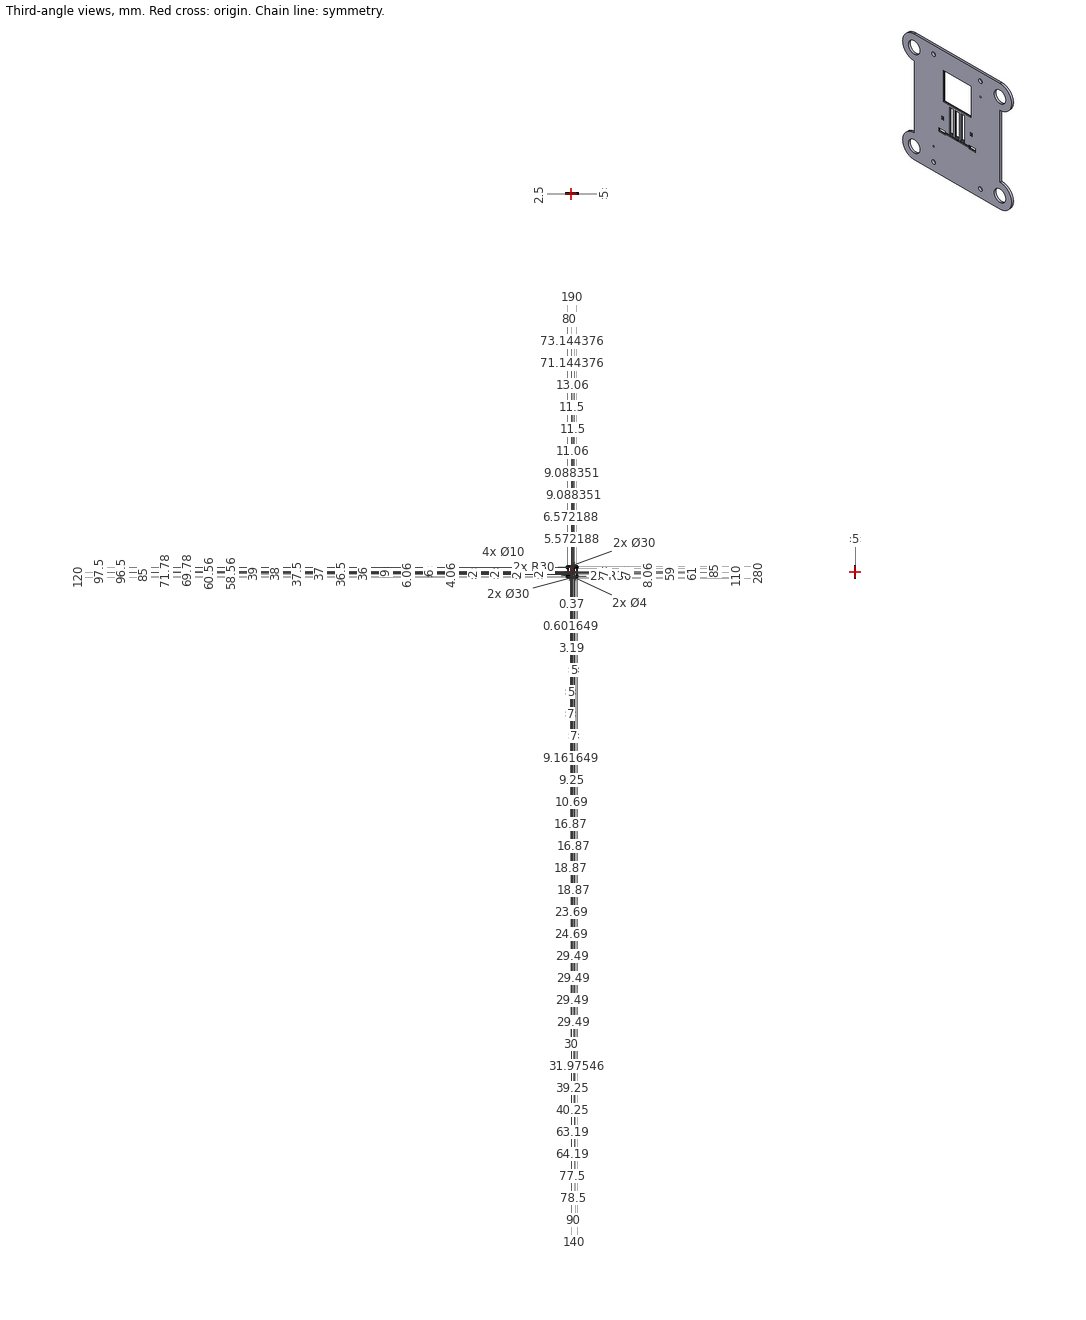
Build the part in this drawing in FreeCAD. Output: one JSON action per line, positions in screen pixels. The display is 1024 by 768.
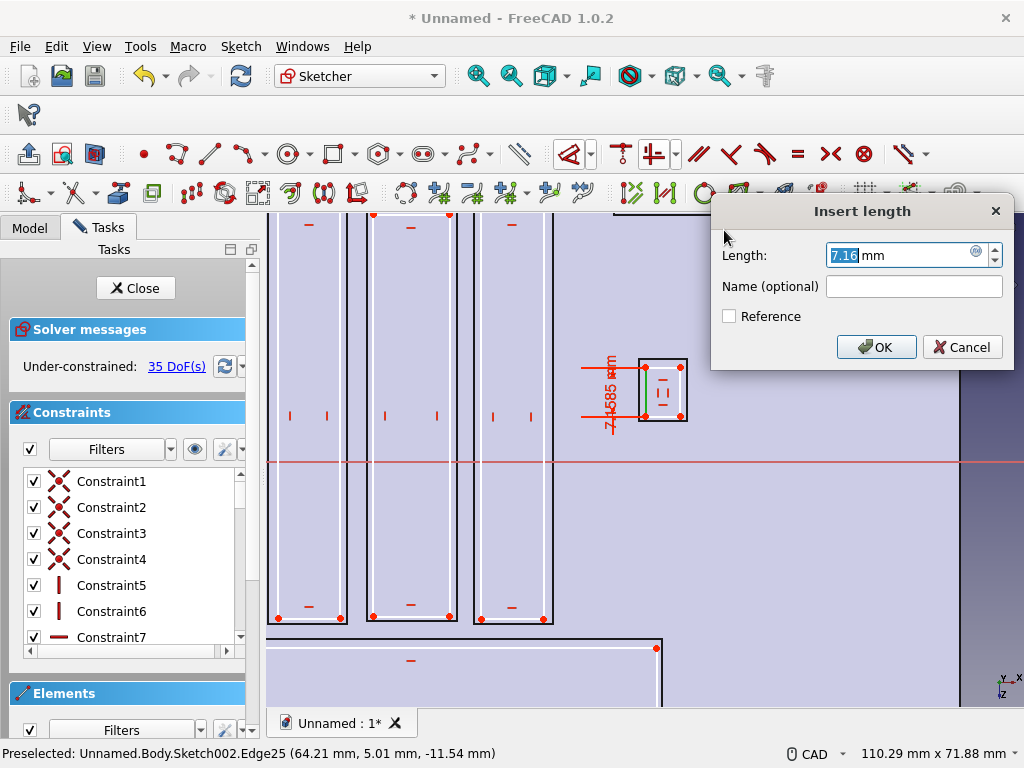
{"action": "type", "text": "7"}
{"action": "key", "text": "Return"}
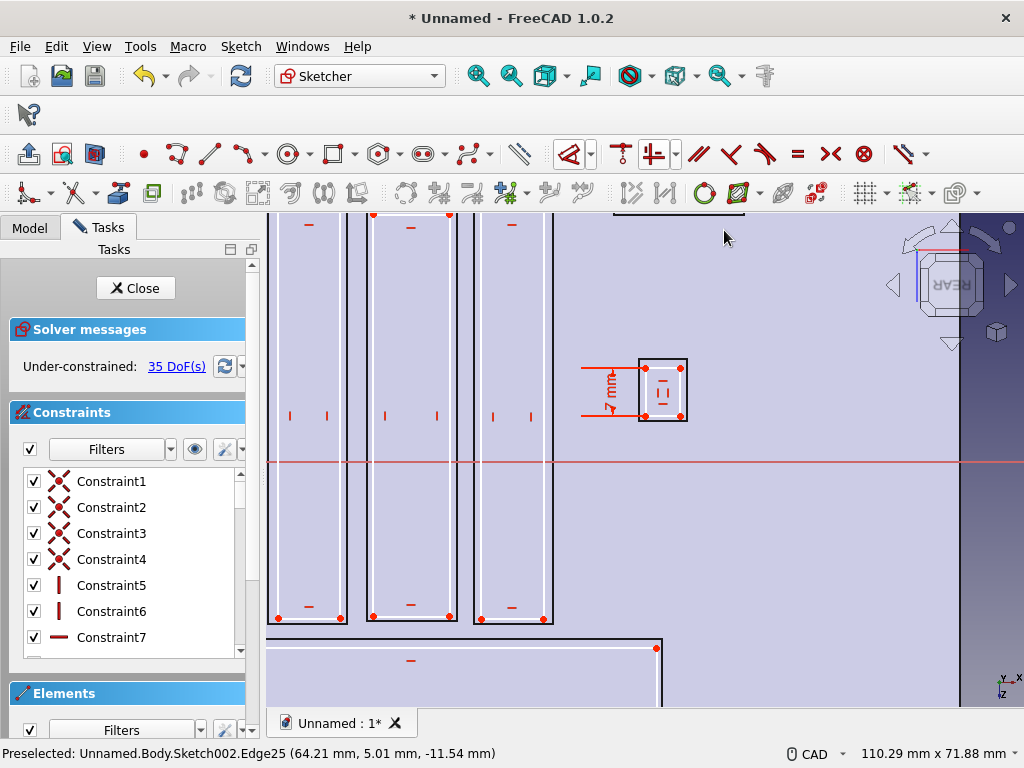
{"action": "scroll", "coordinate": [656, 416], "scroll_direction": "up", "scroll_amount": 2}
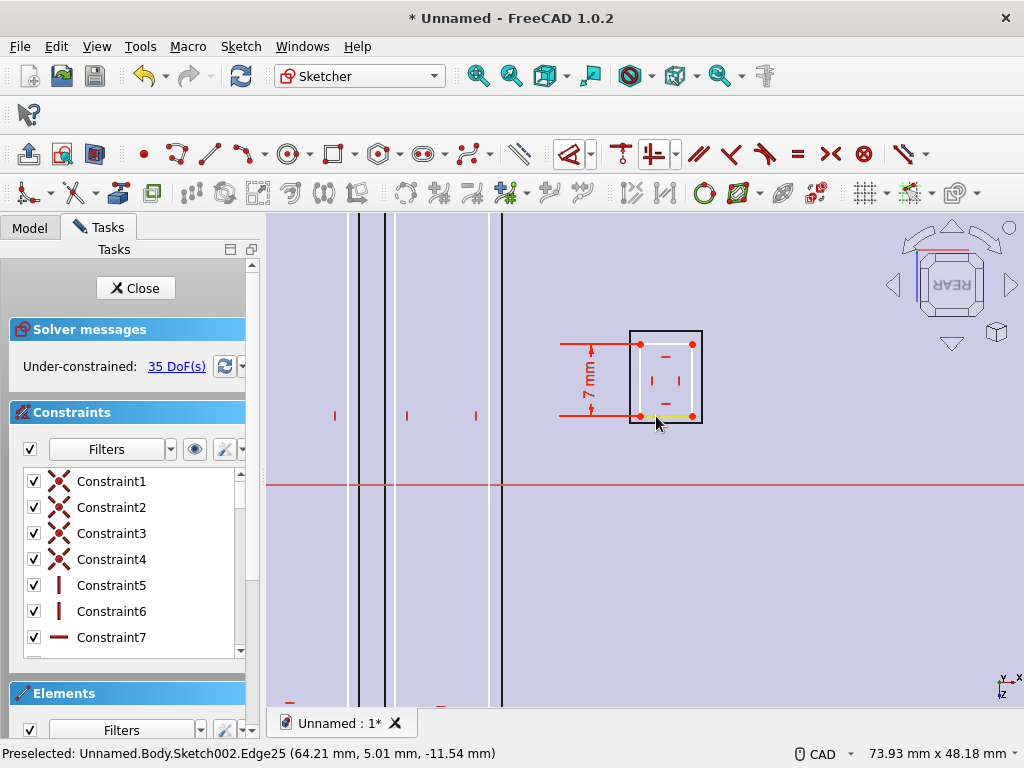
{"action": "left_click", "coordinate": [656, 416]}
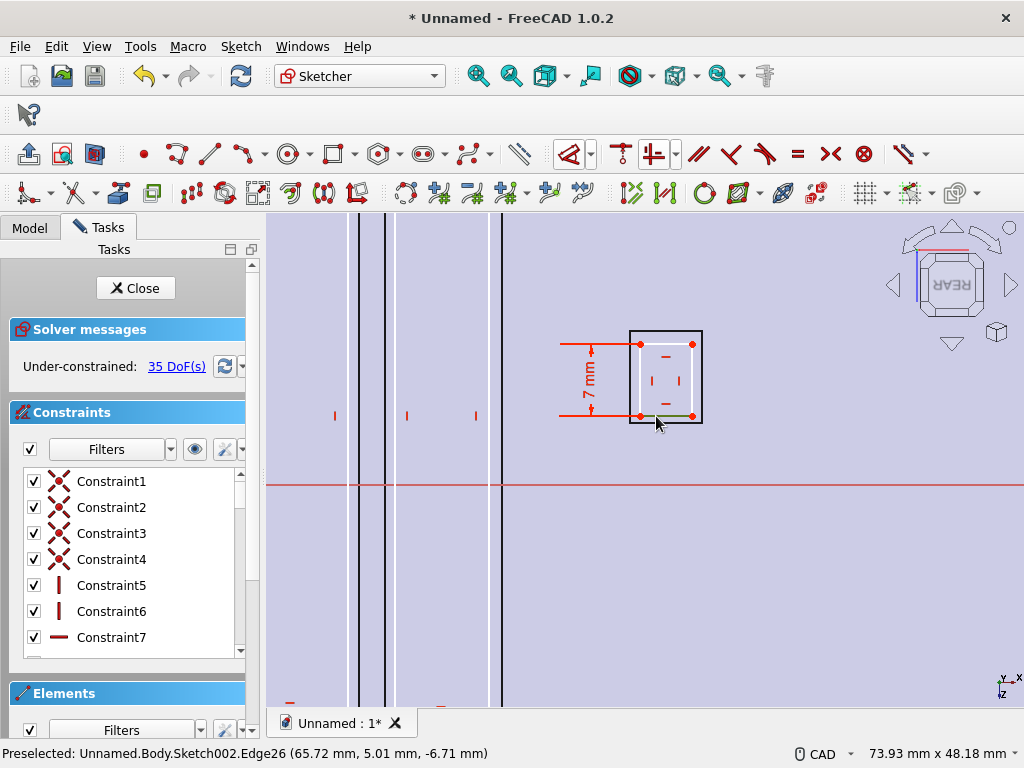
{"action": "left_click", "coordinate": [590, 154]}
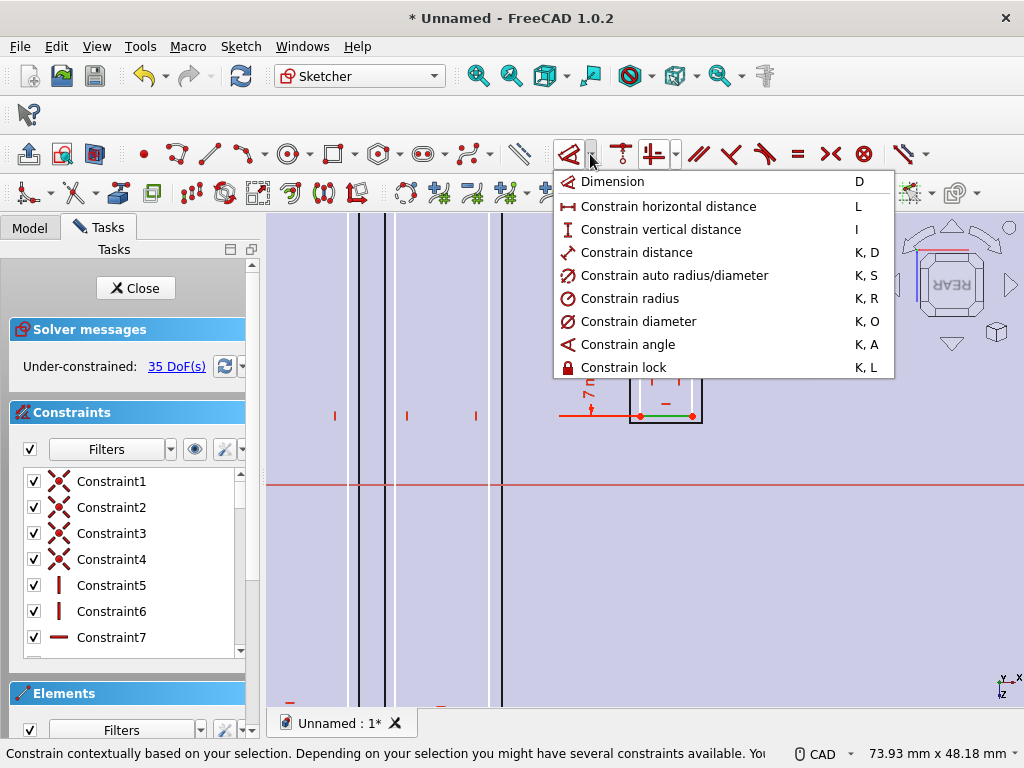
{"action": "left_click", "coordinate": [724, 206]}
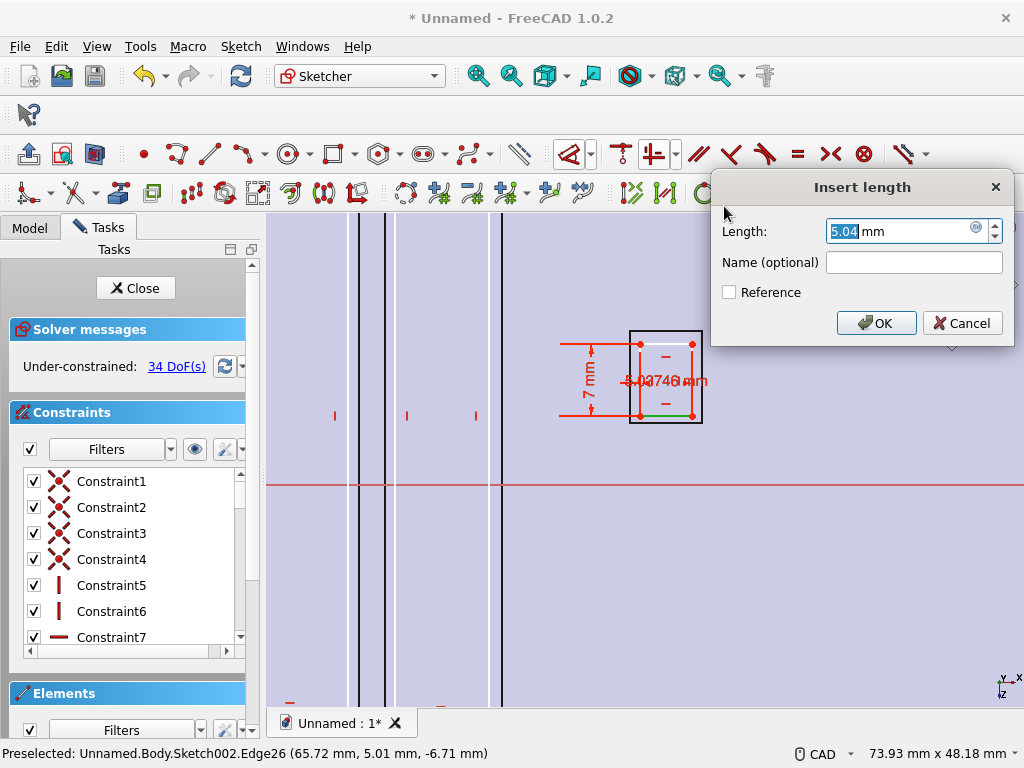
{"action": "type", "text": "5"}
{"action": "key", "text": "Return"}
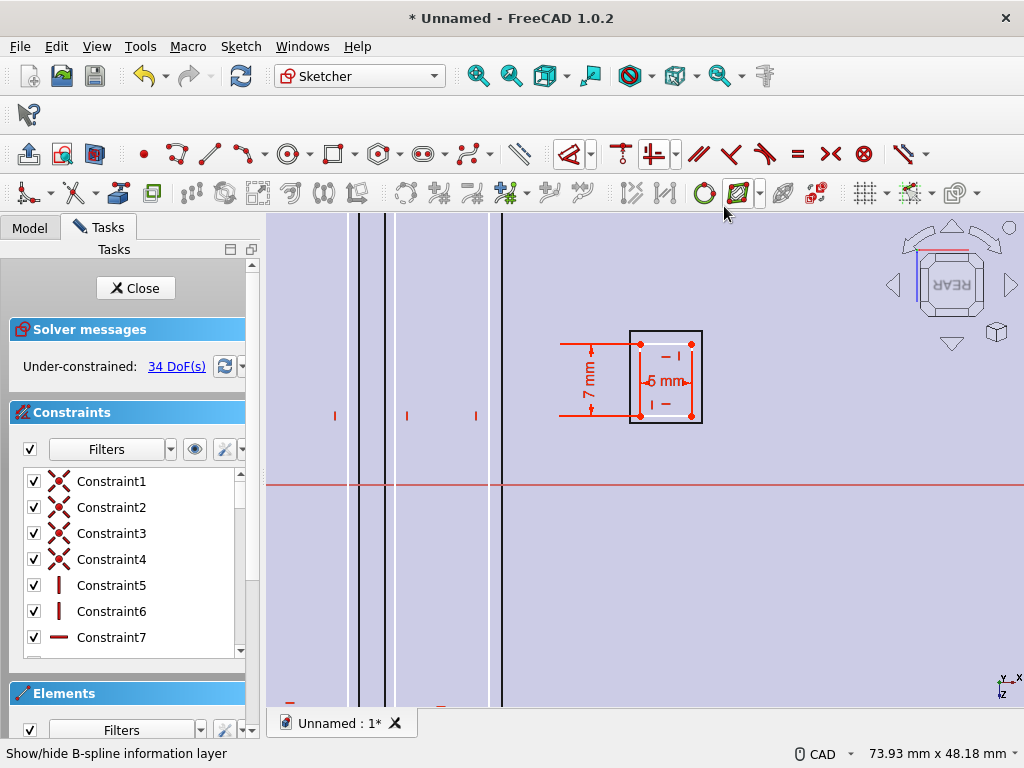
{"action": "scroll", "coordinate": [649, 387], "scroll_direction": "down", "scroll_amount": 8}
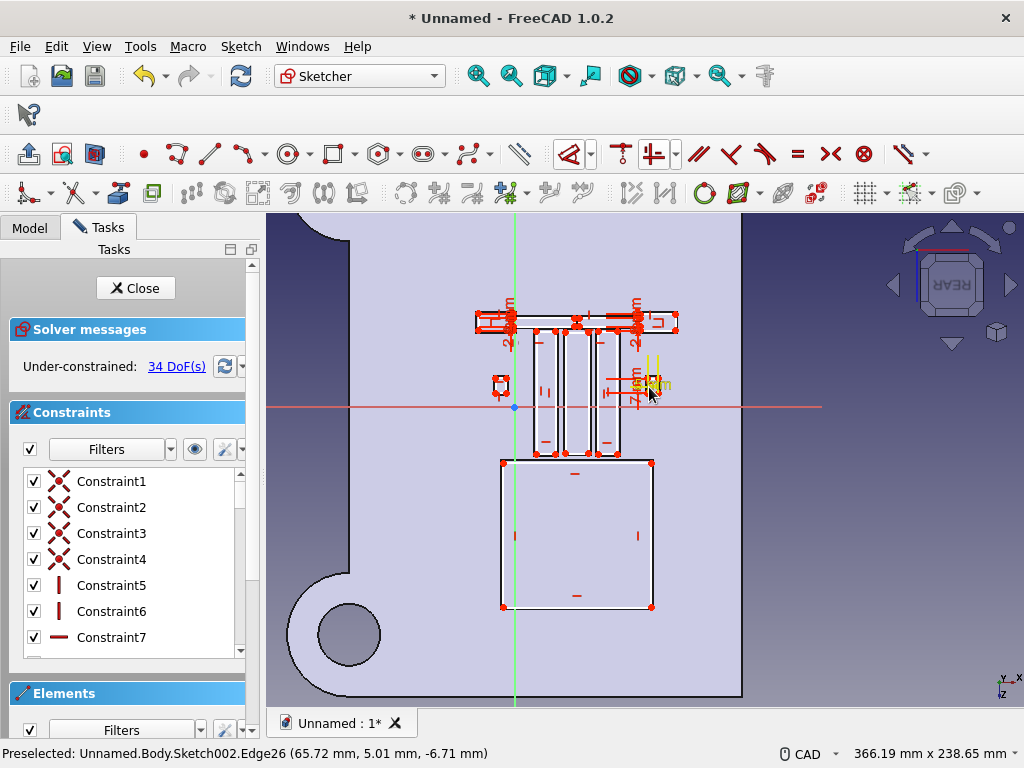
{"action": "scroll", "coordinate": [496, 383], "scroll_direction": "up", "scroll_amount": 6}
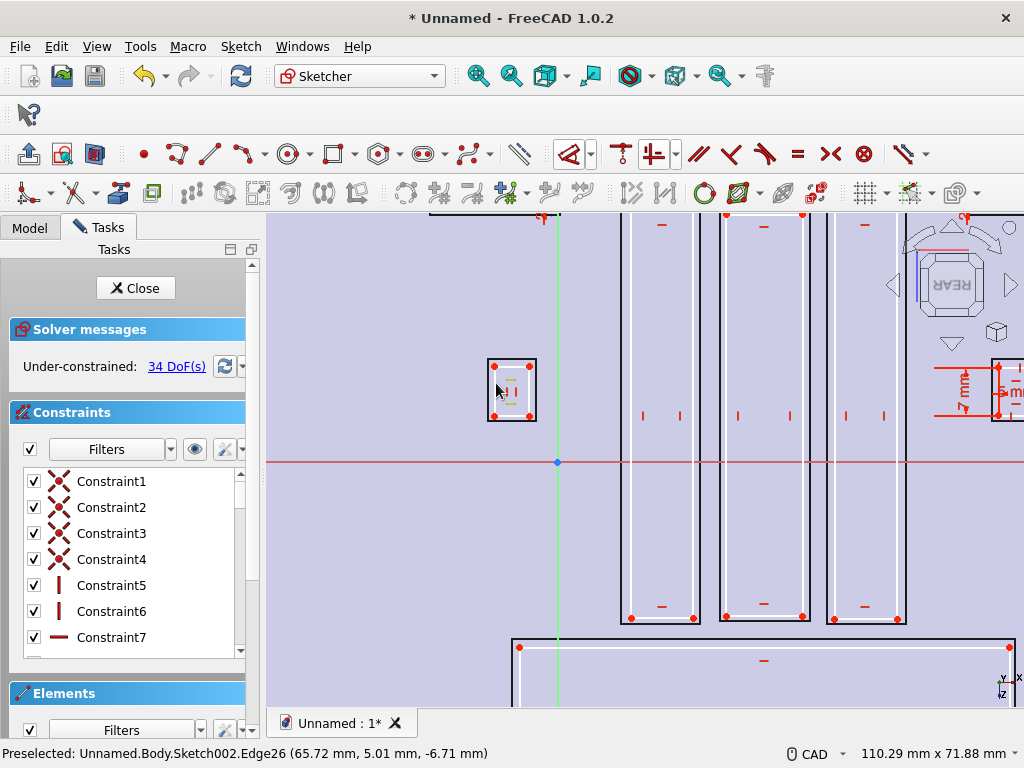
{"action": "left_click", "coordinate": [495, 382]}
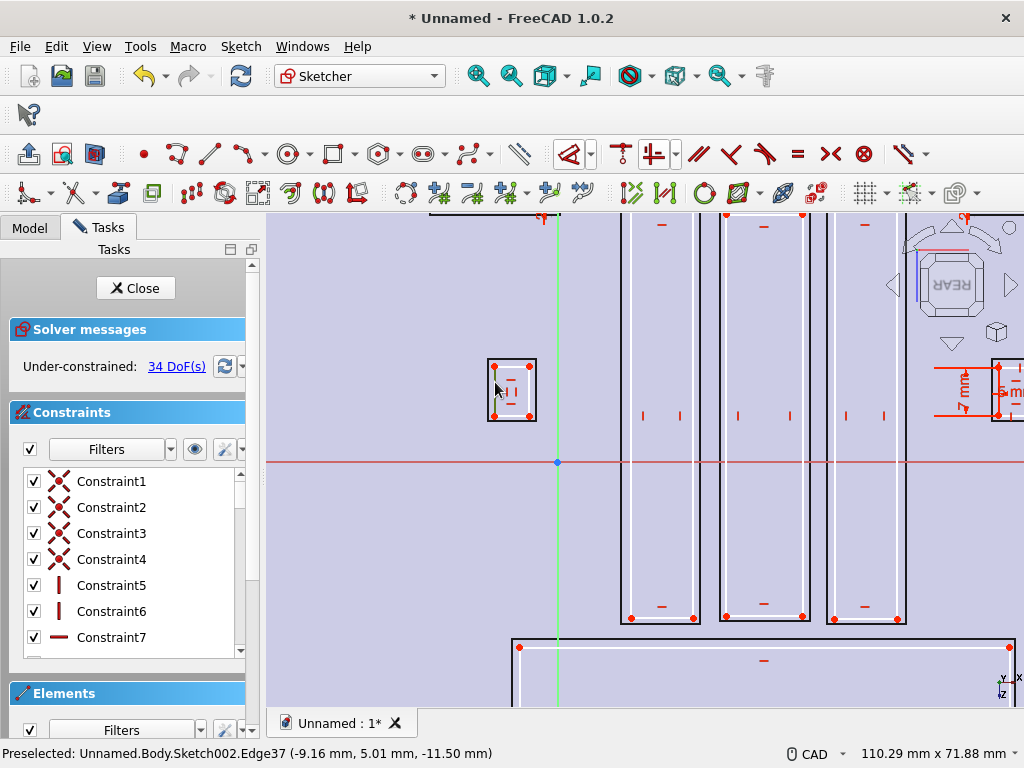
{"action": "left_click", "coordinate": [590, 154]}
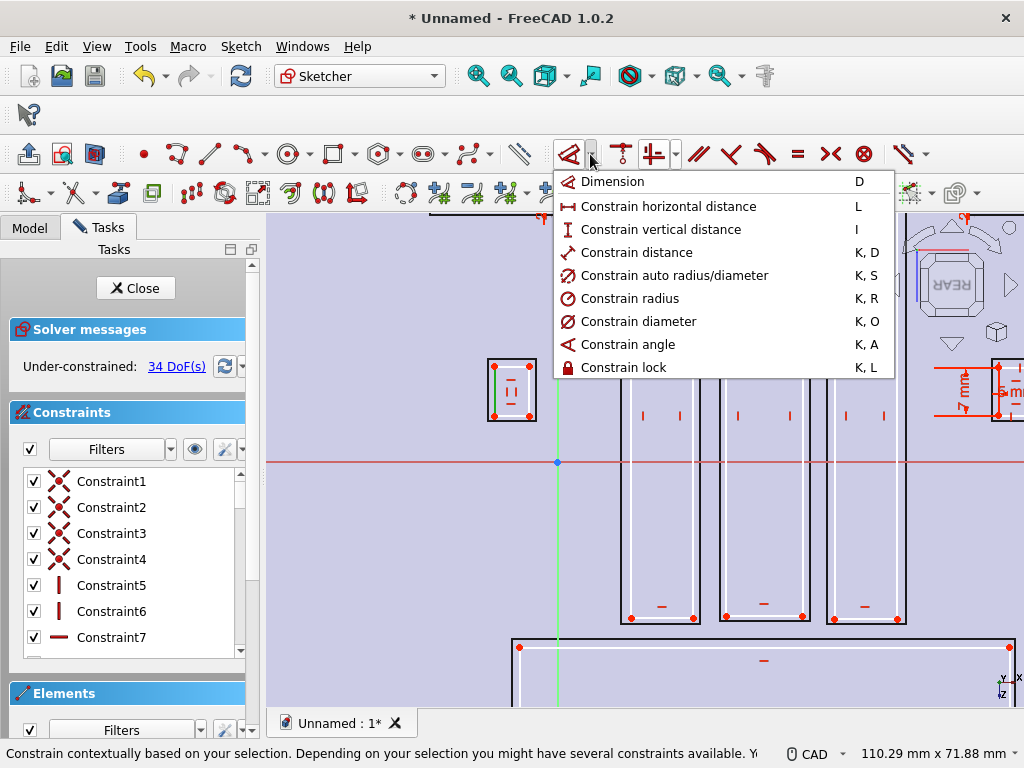
{"action": "left_click", "coordinate": [724, 230]}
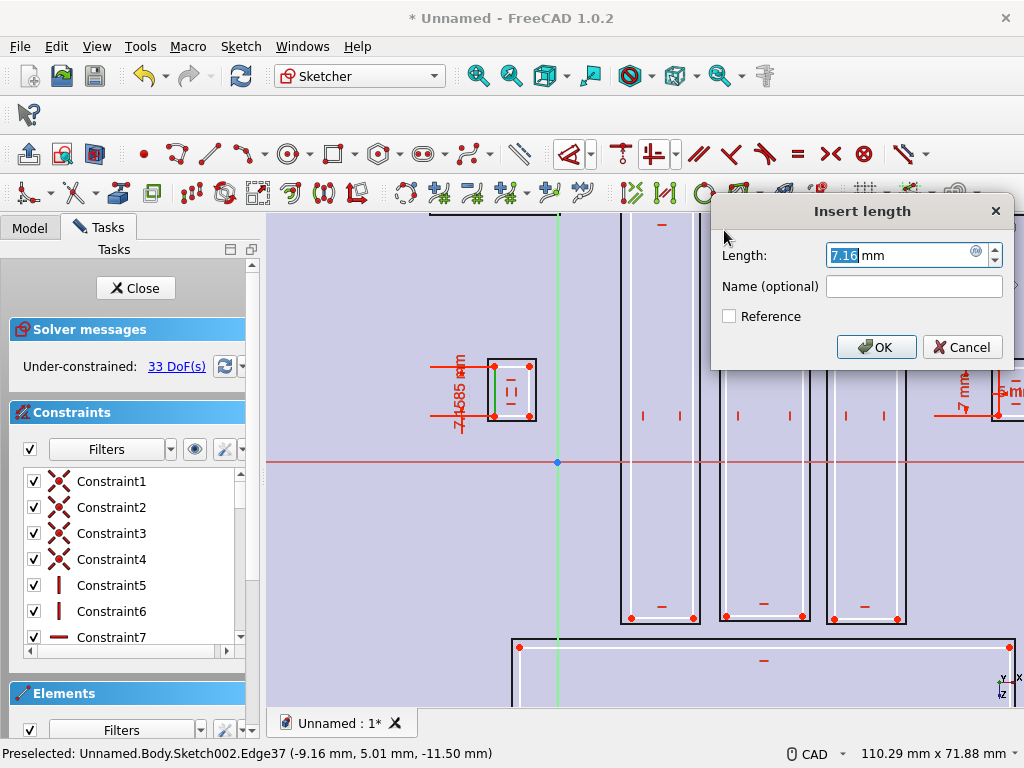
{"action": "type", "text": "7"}
{"action": "key", "text": "Return"}